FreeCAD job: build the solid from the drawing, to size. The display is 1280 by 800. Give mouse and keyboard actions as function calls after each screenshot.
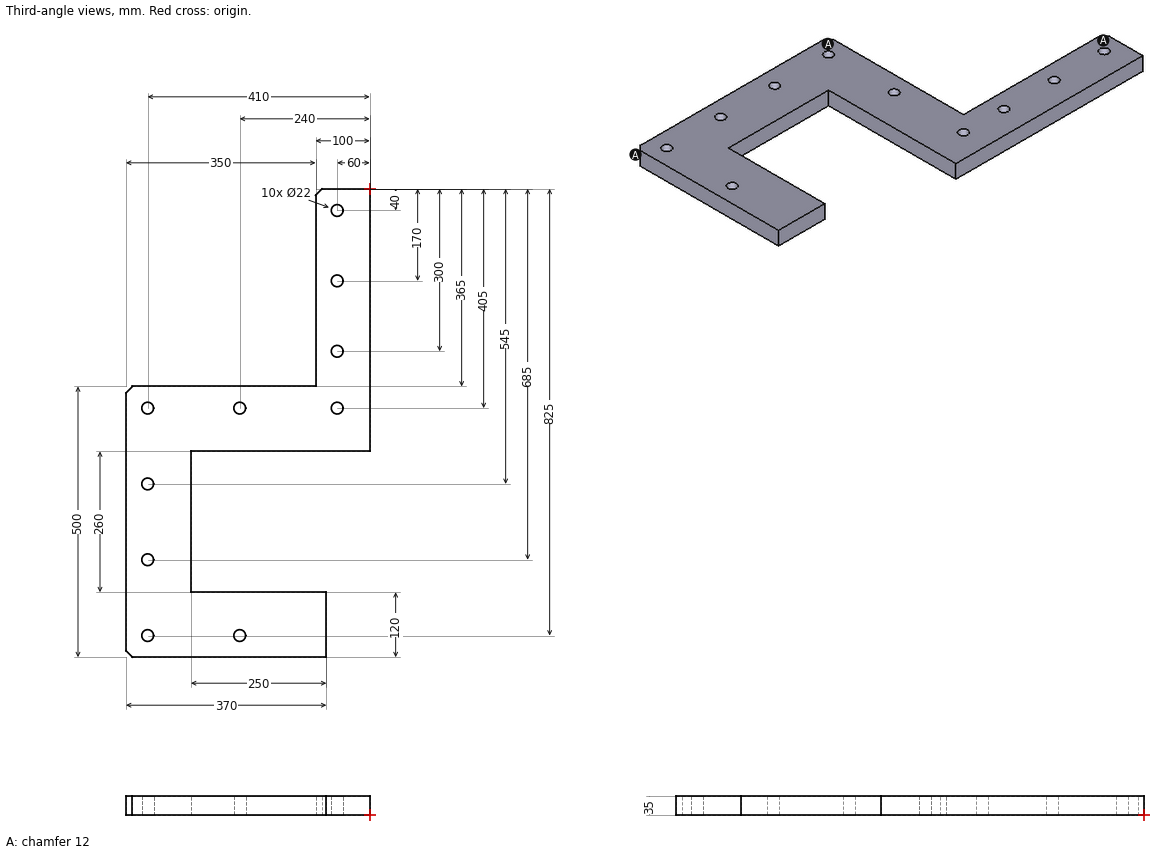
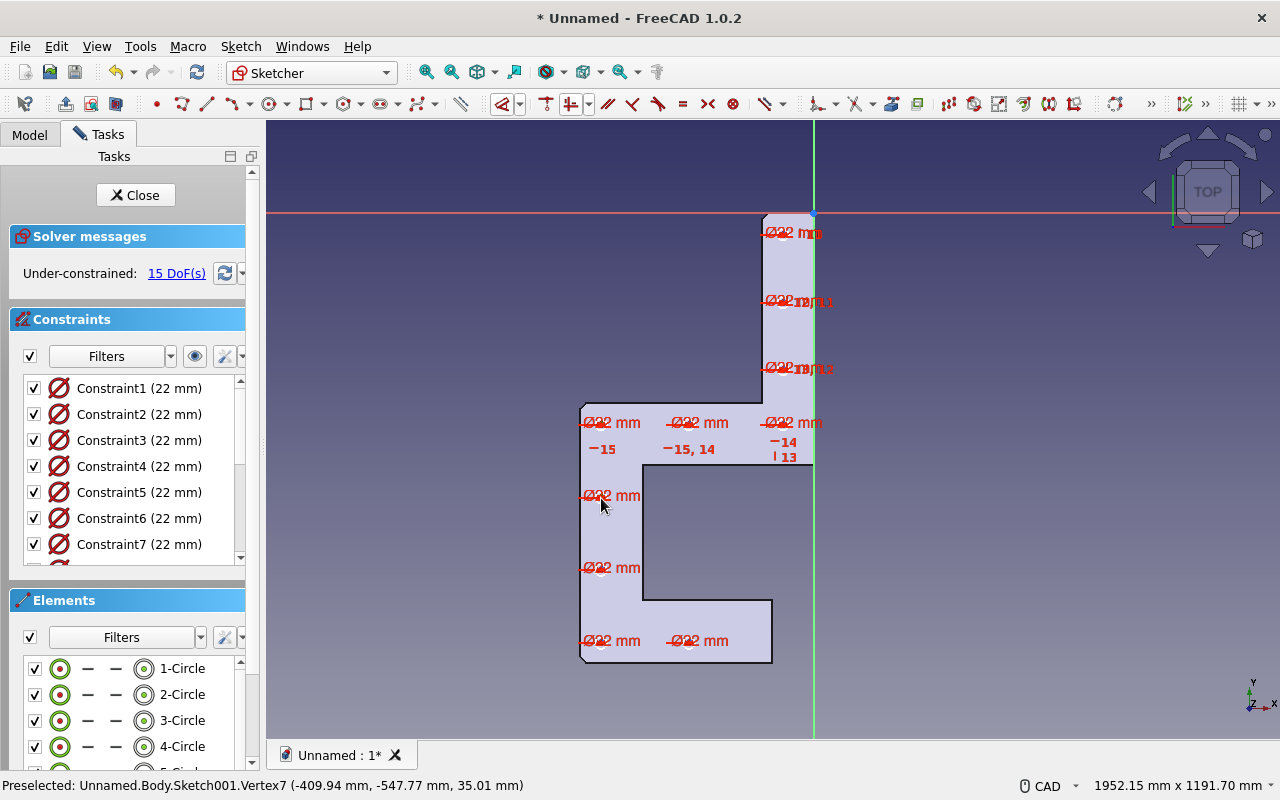
click(588, 104)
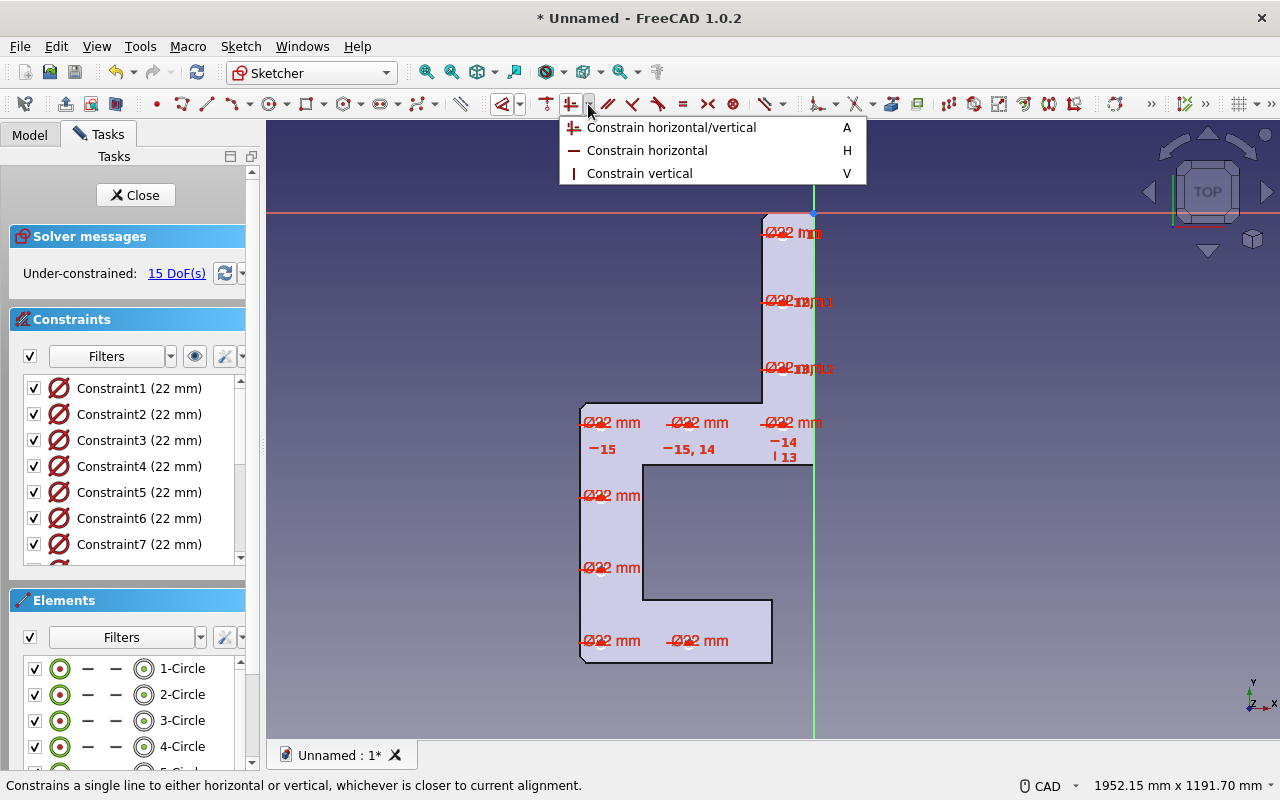
click(713, 174)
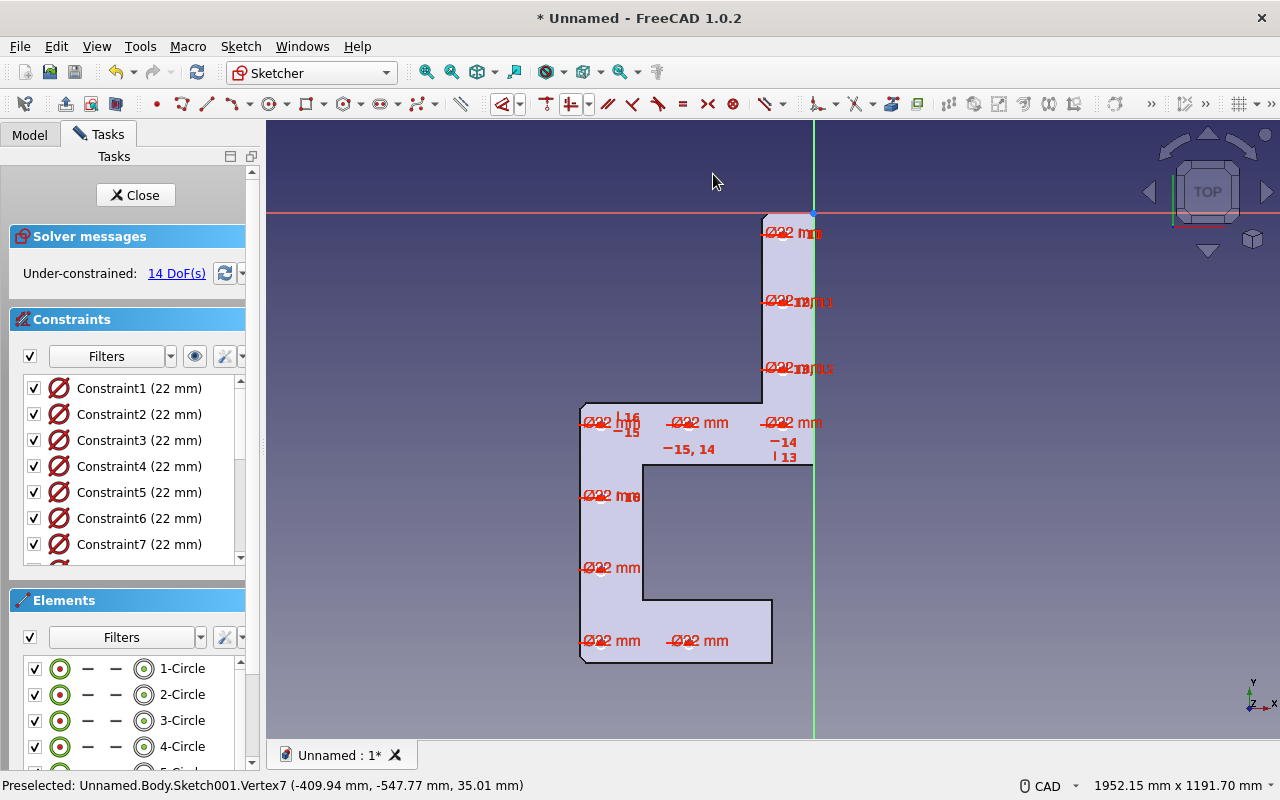
click(601, 498)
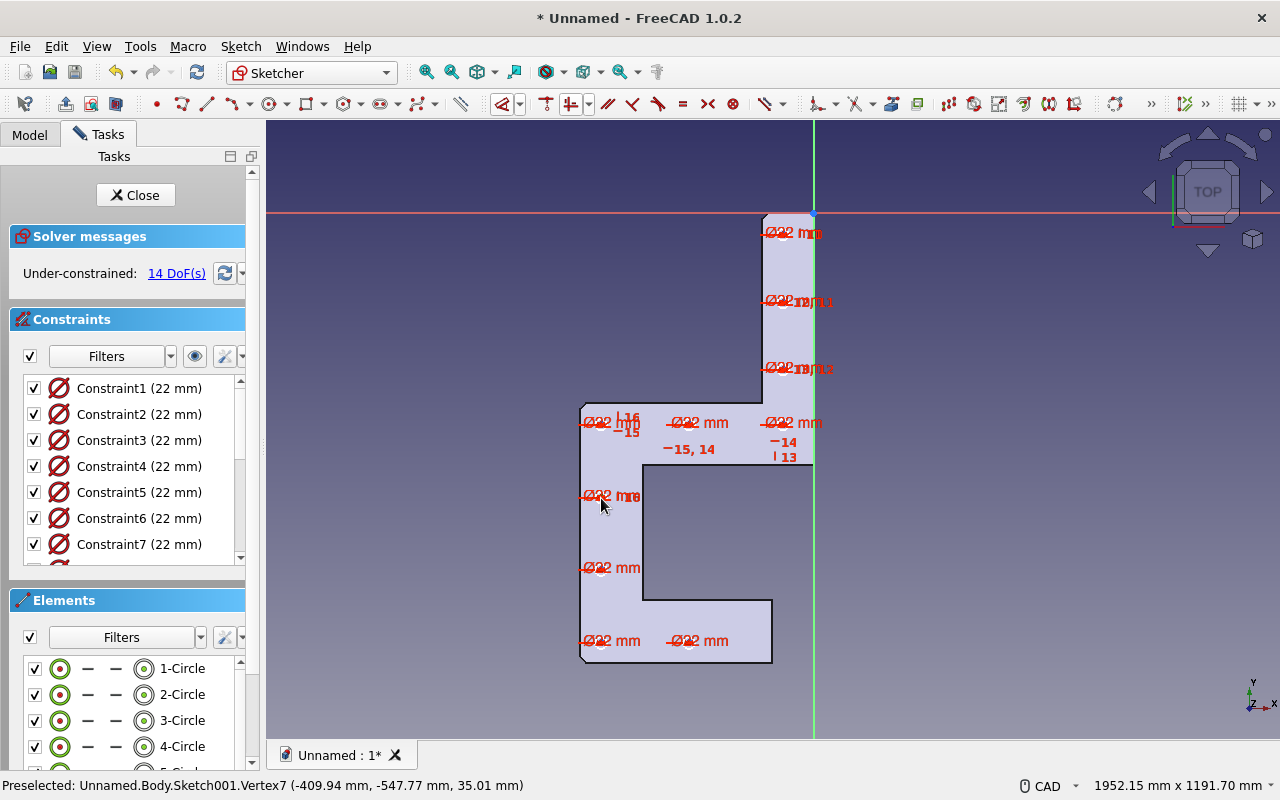
click(601, 570)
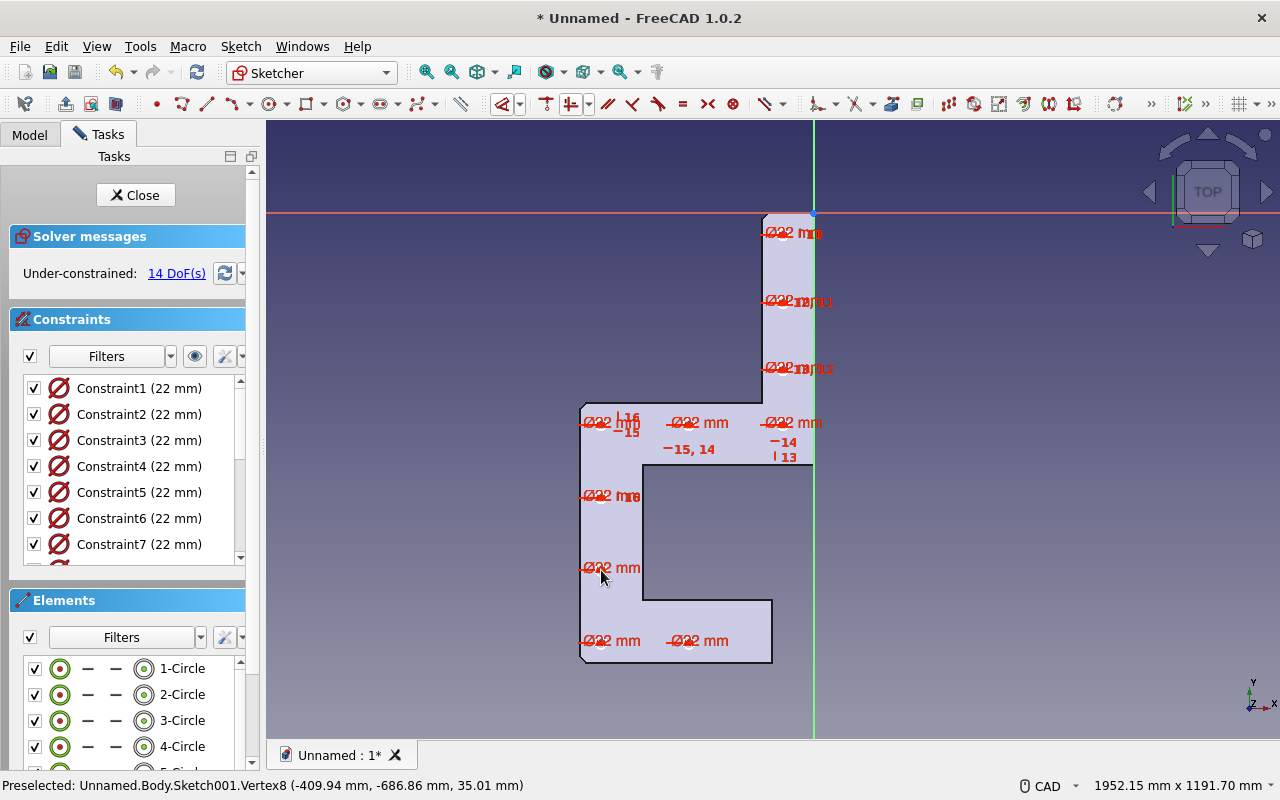
key(v)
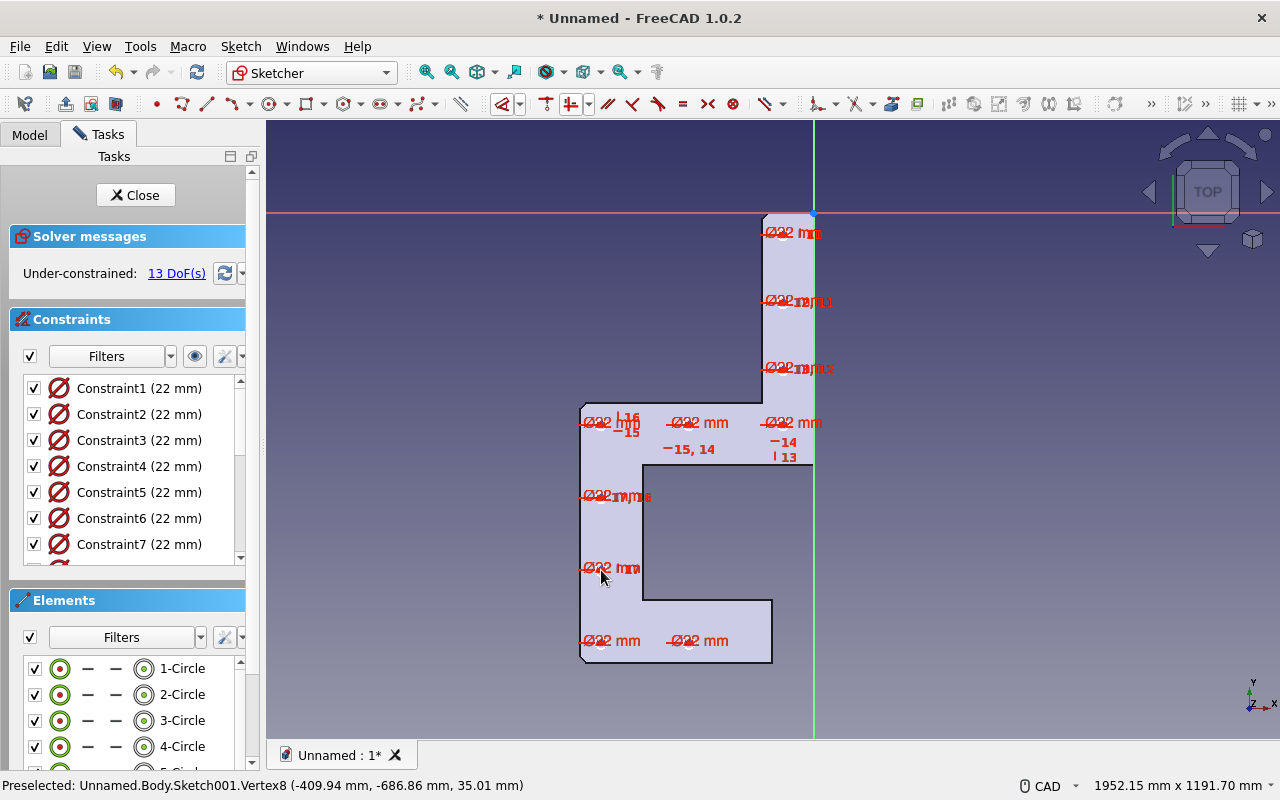
click(601, 570)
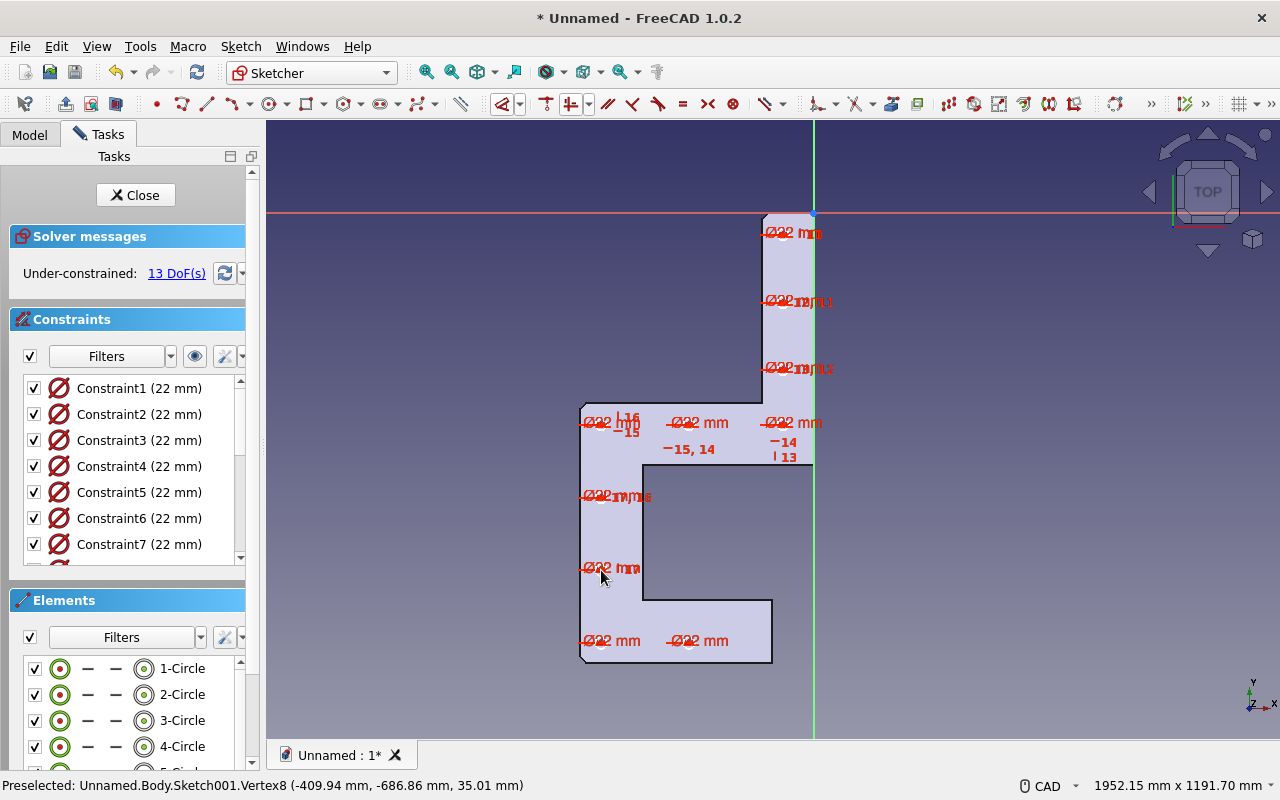
click(601, 643)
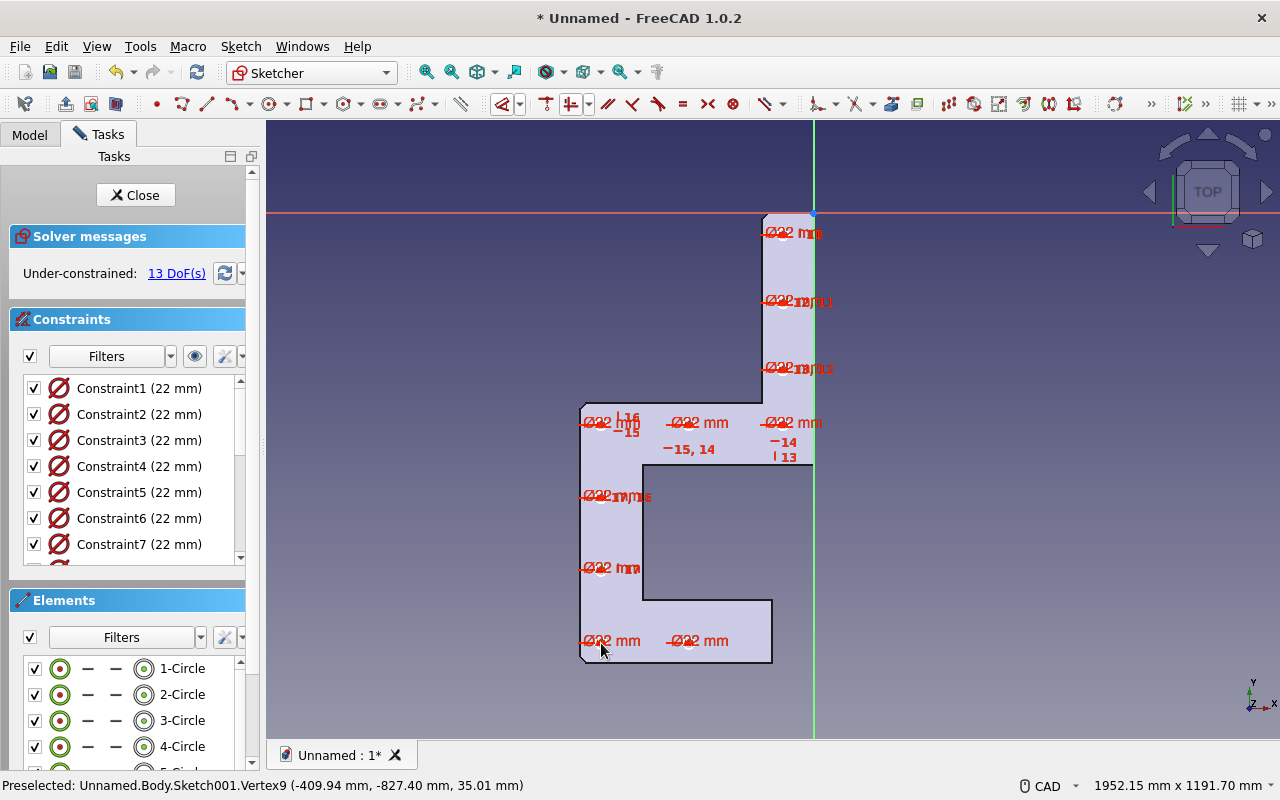
key(v)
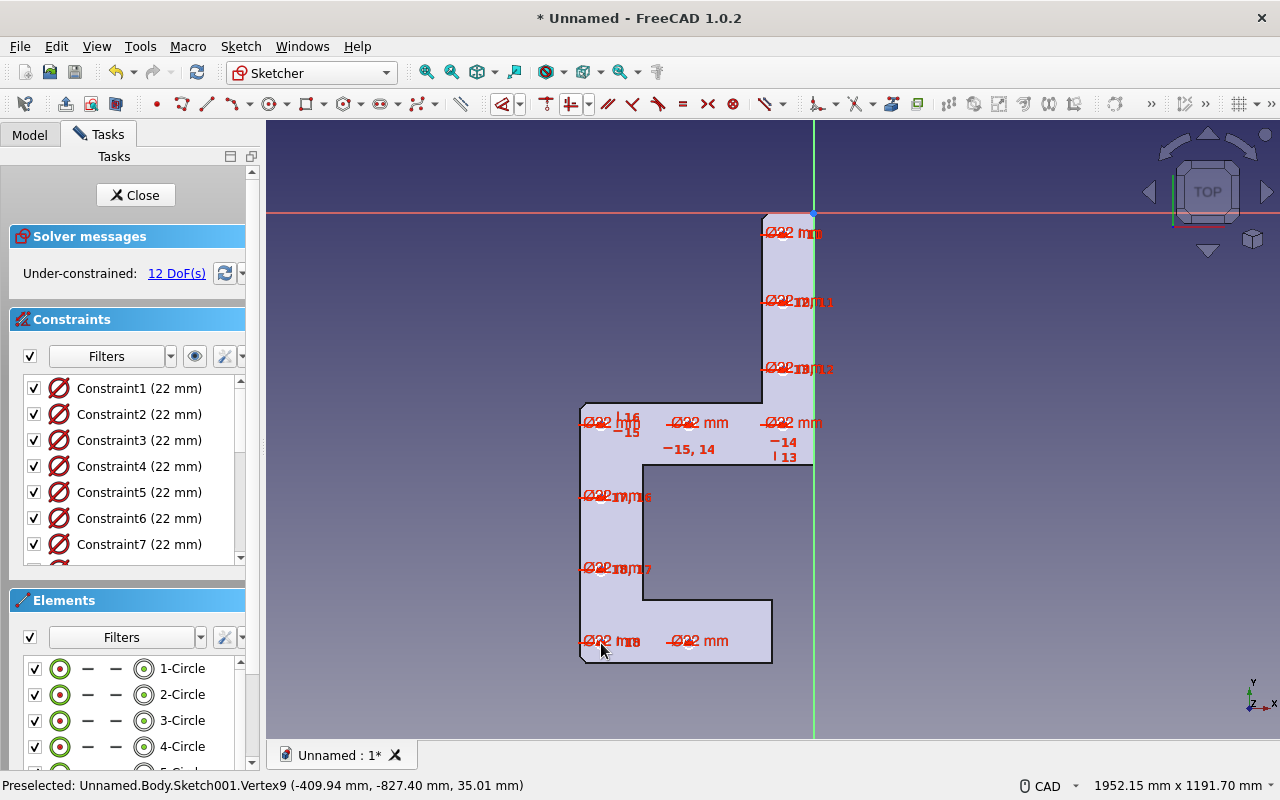
click(689, 425)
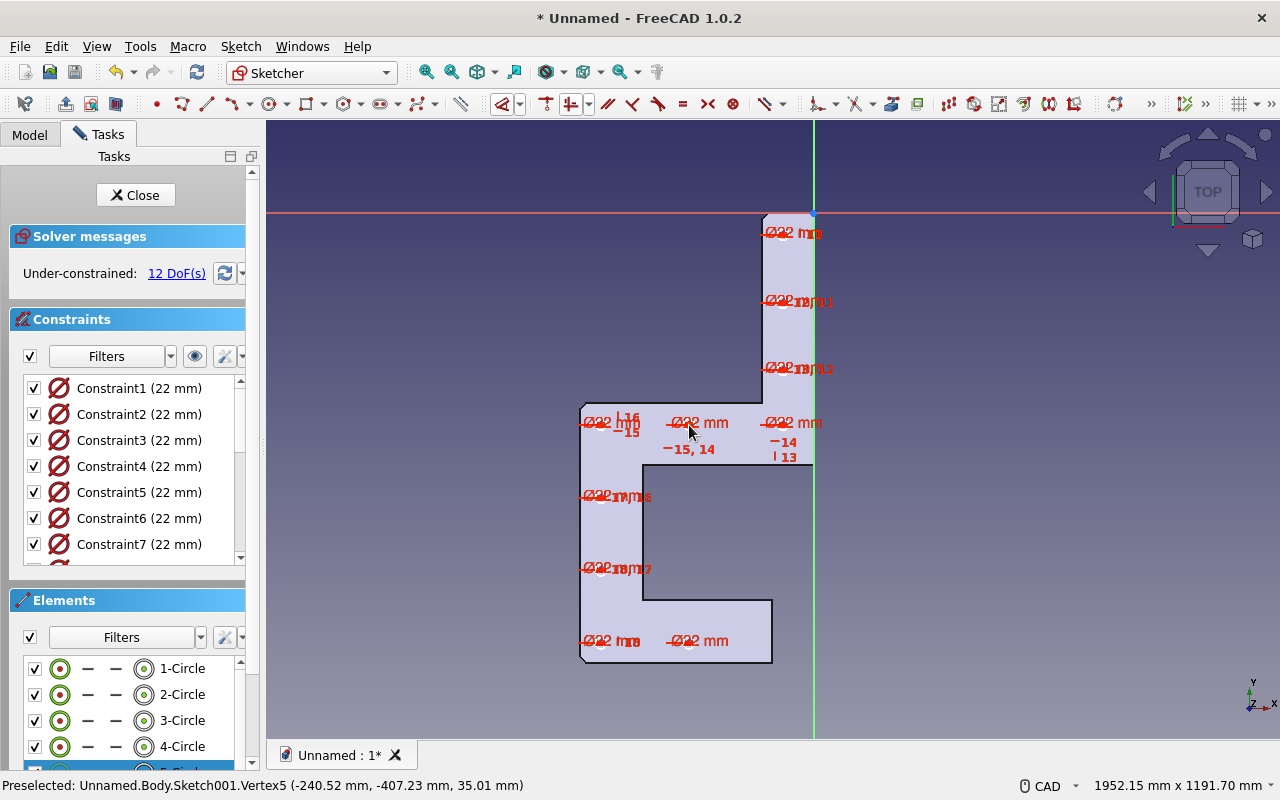
click(689, 643)